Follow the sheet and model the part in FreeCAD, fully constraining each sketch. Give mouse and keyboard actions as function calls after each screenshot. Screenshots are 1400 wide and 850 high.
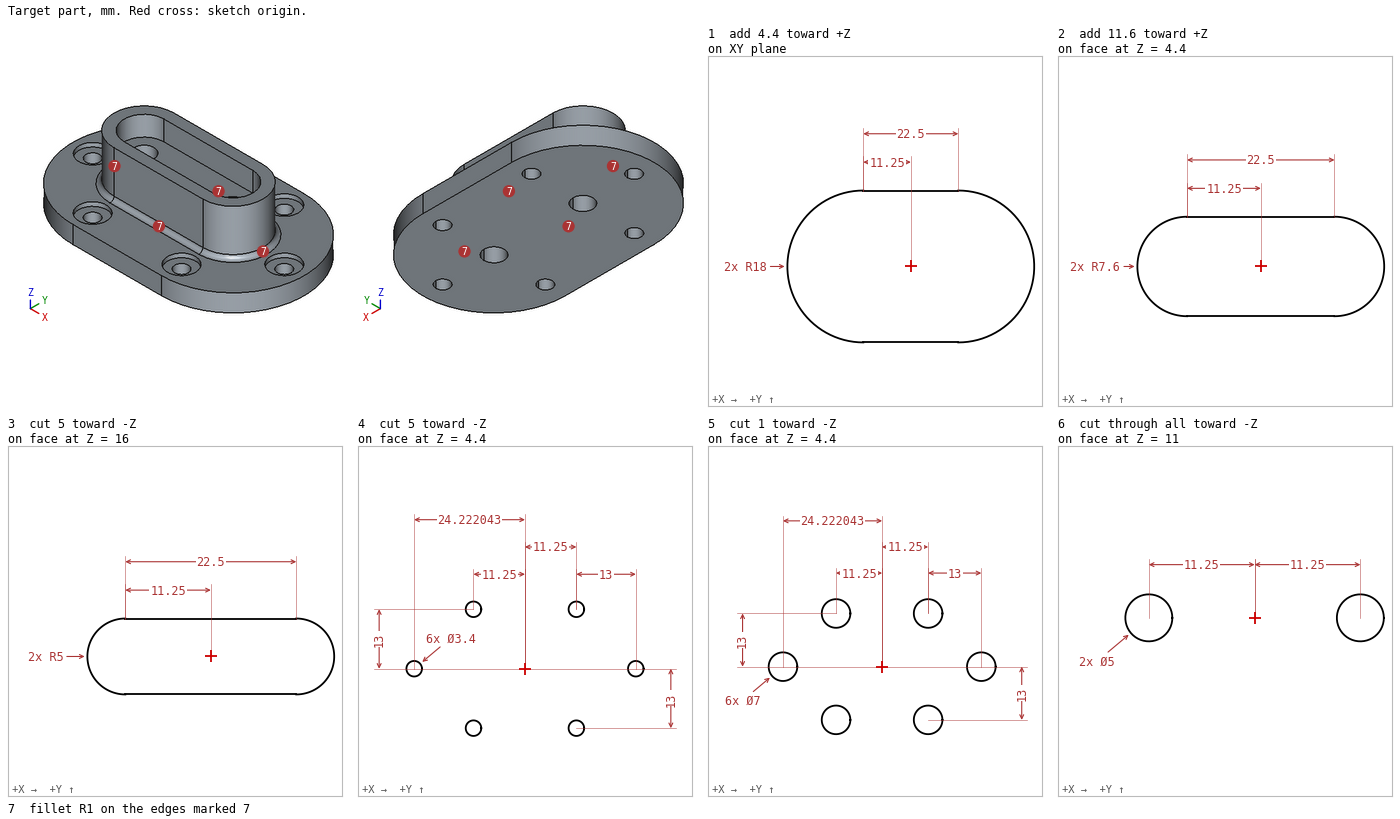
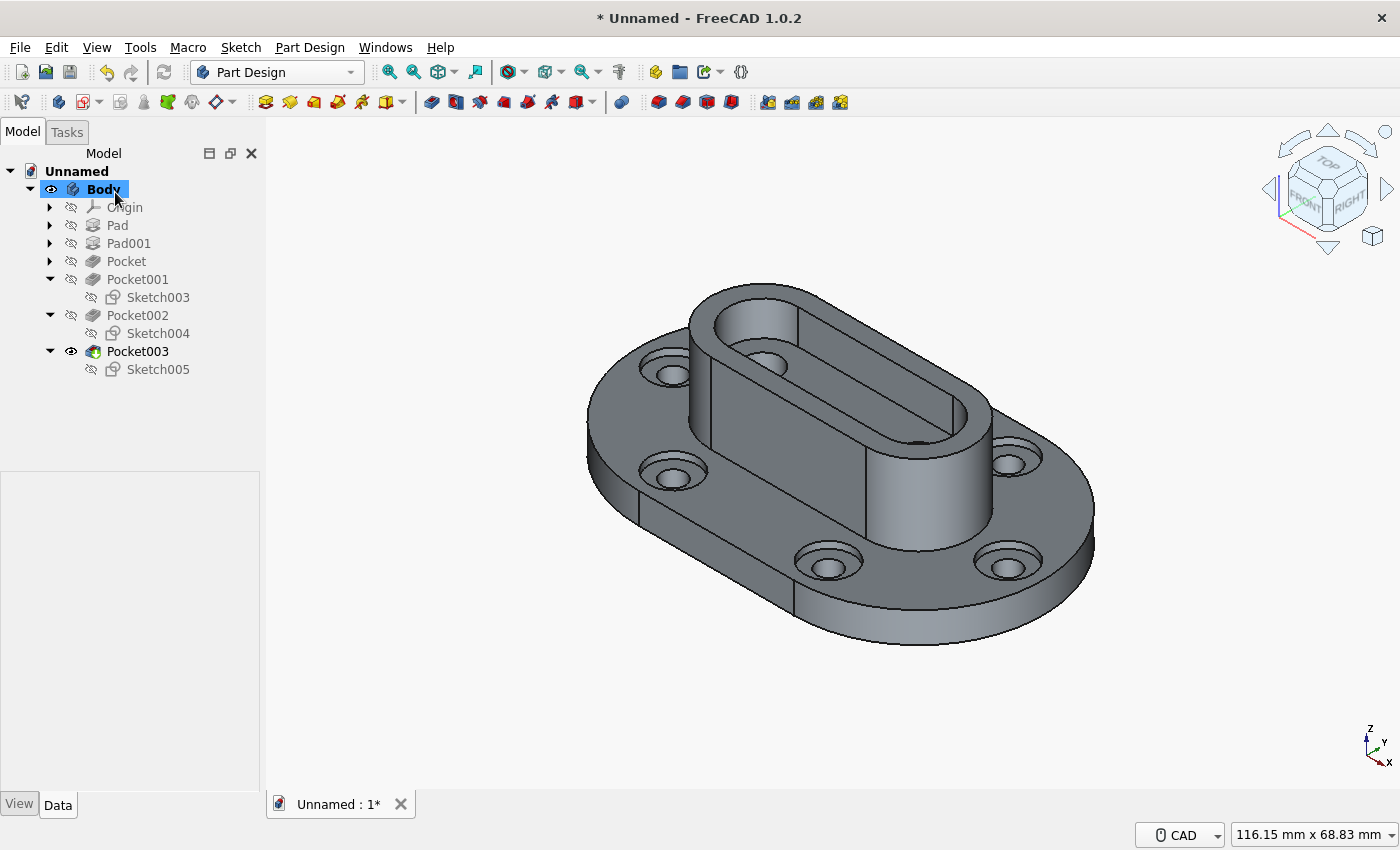
key(2)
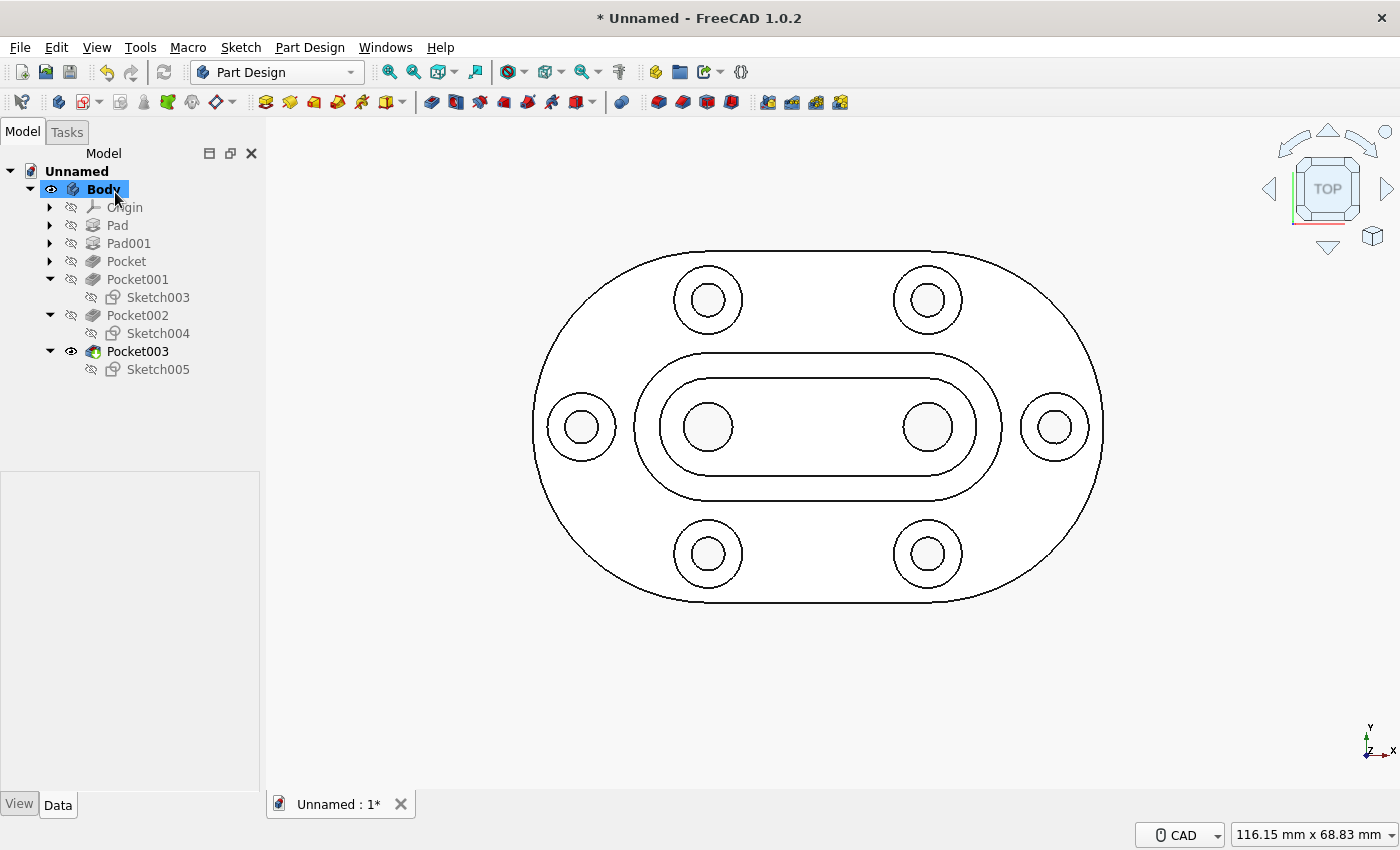
key(1)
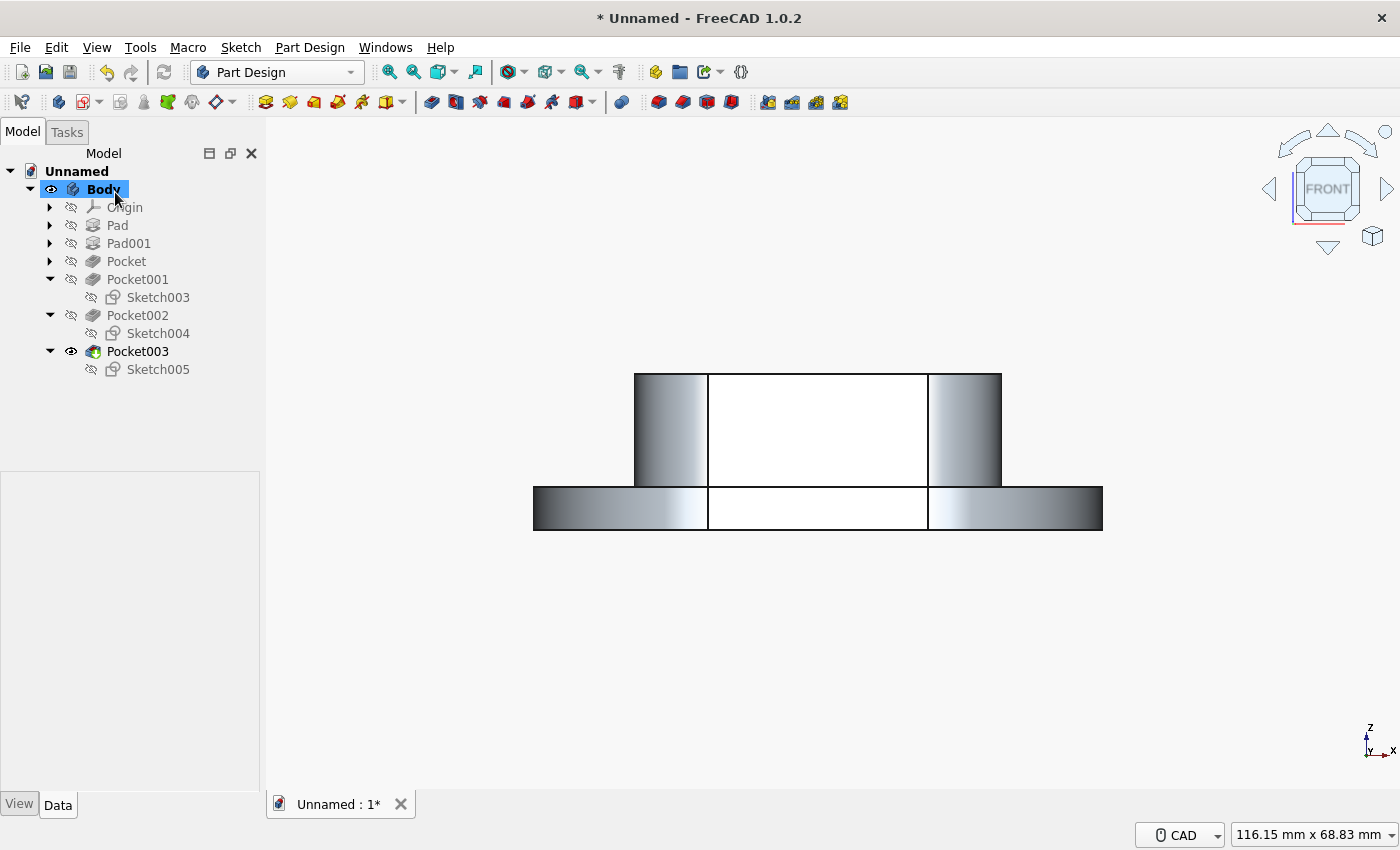
key(3)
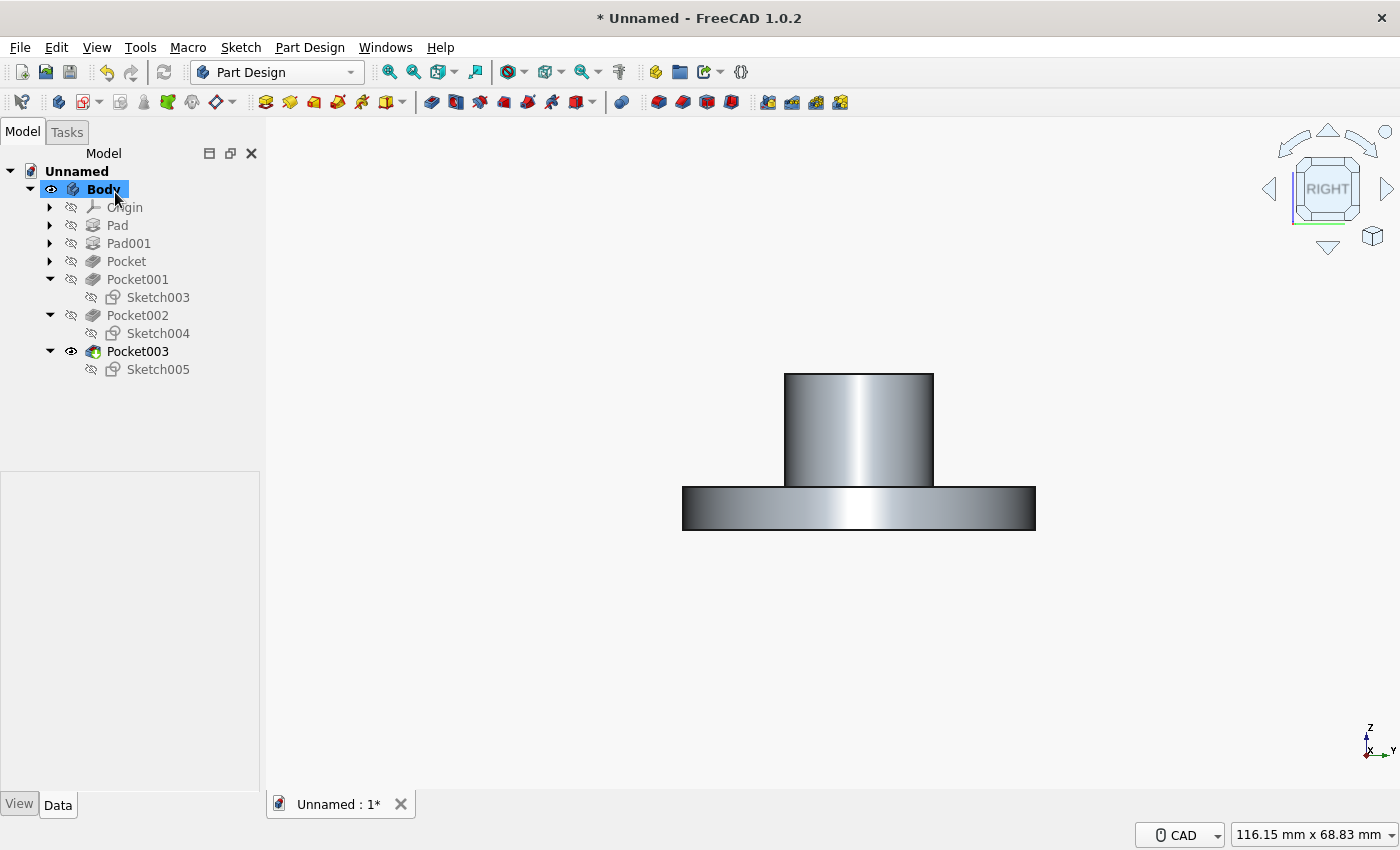
click(390, 72)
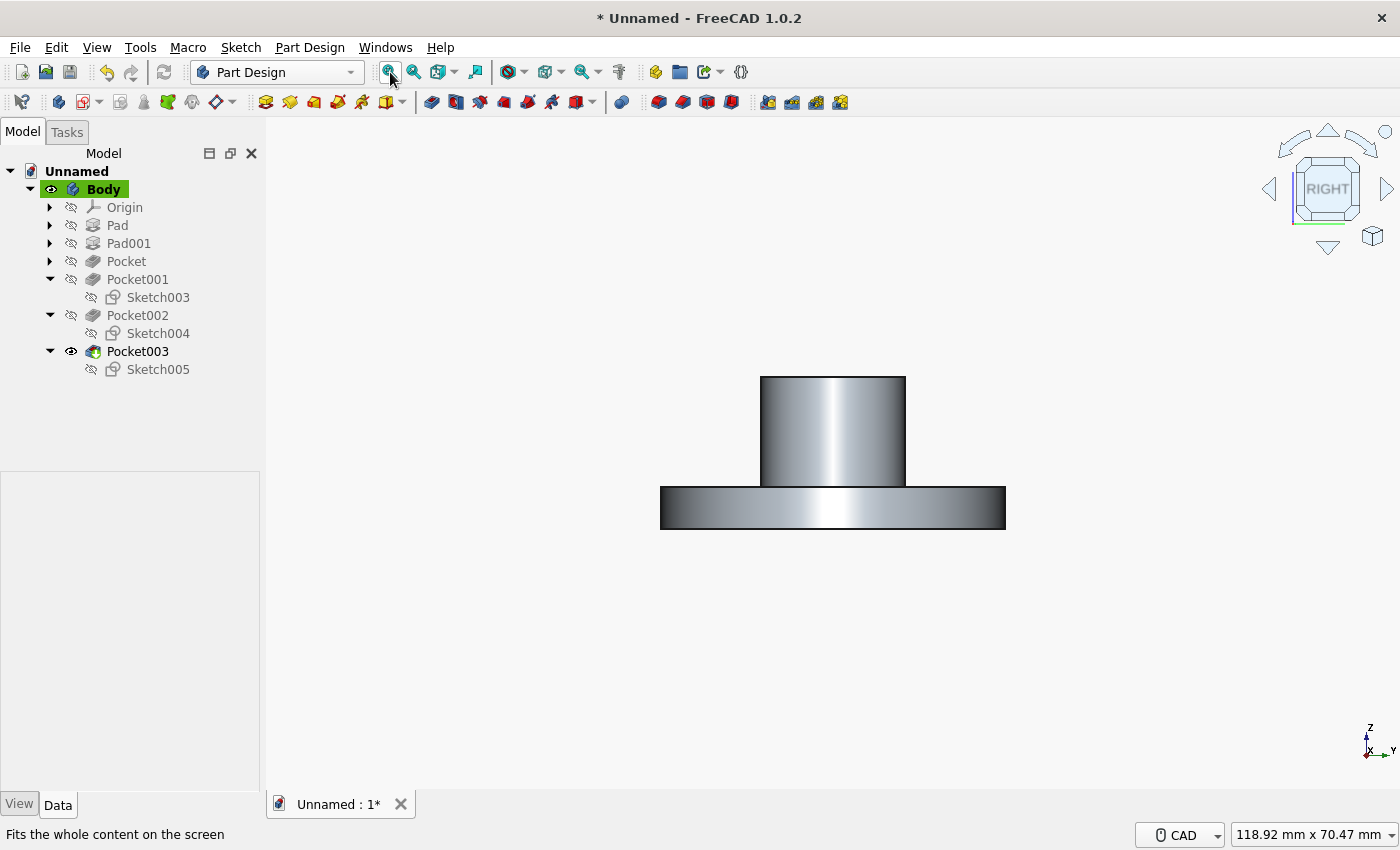
key(5)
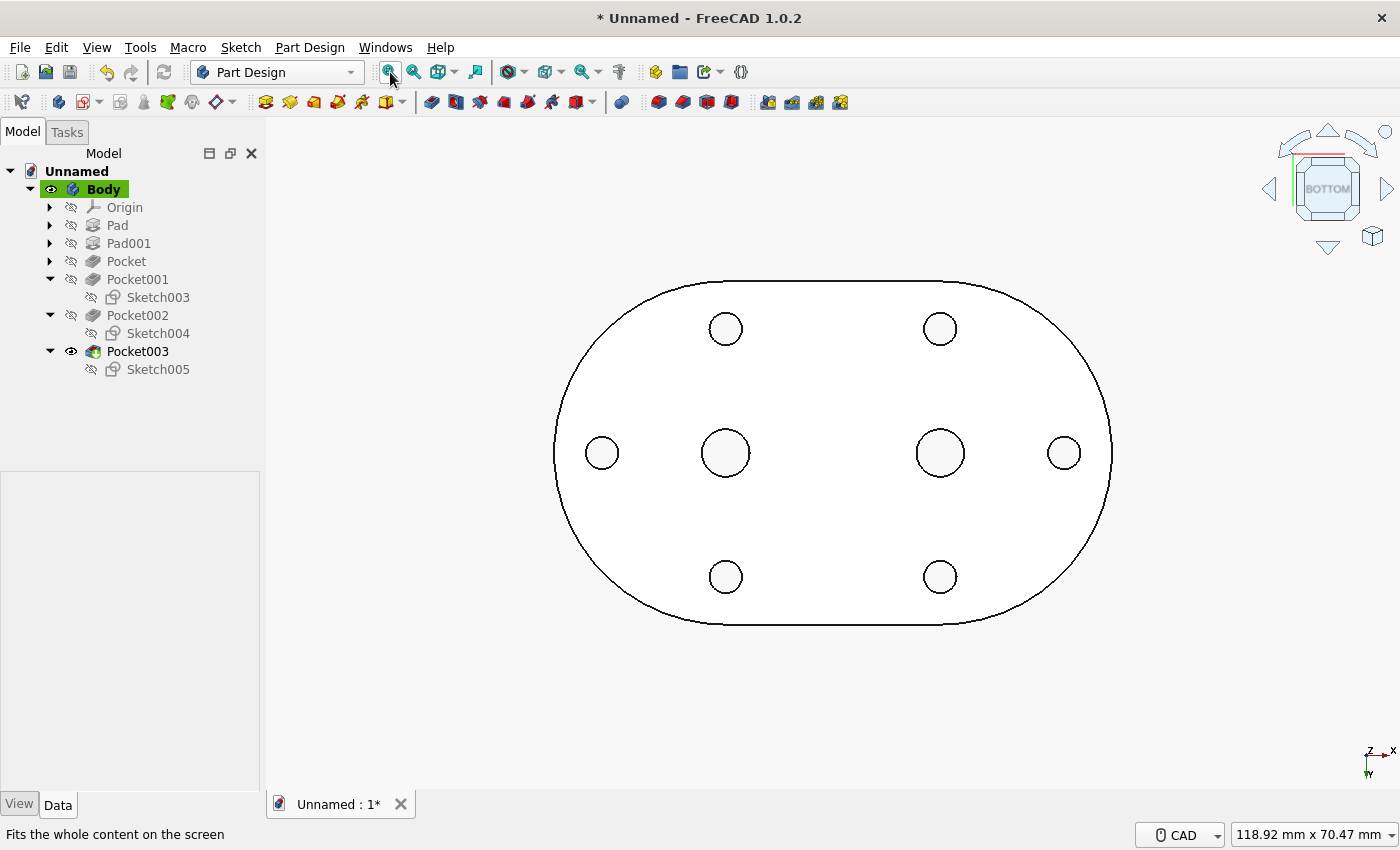
key(4)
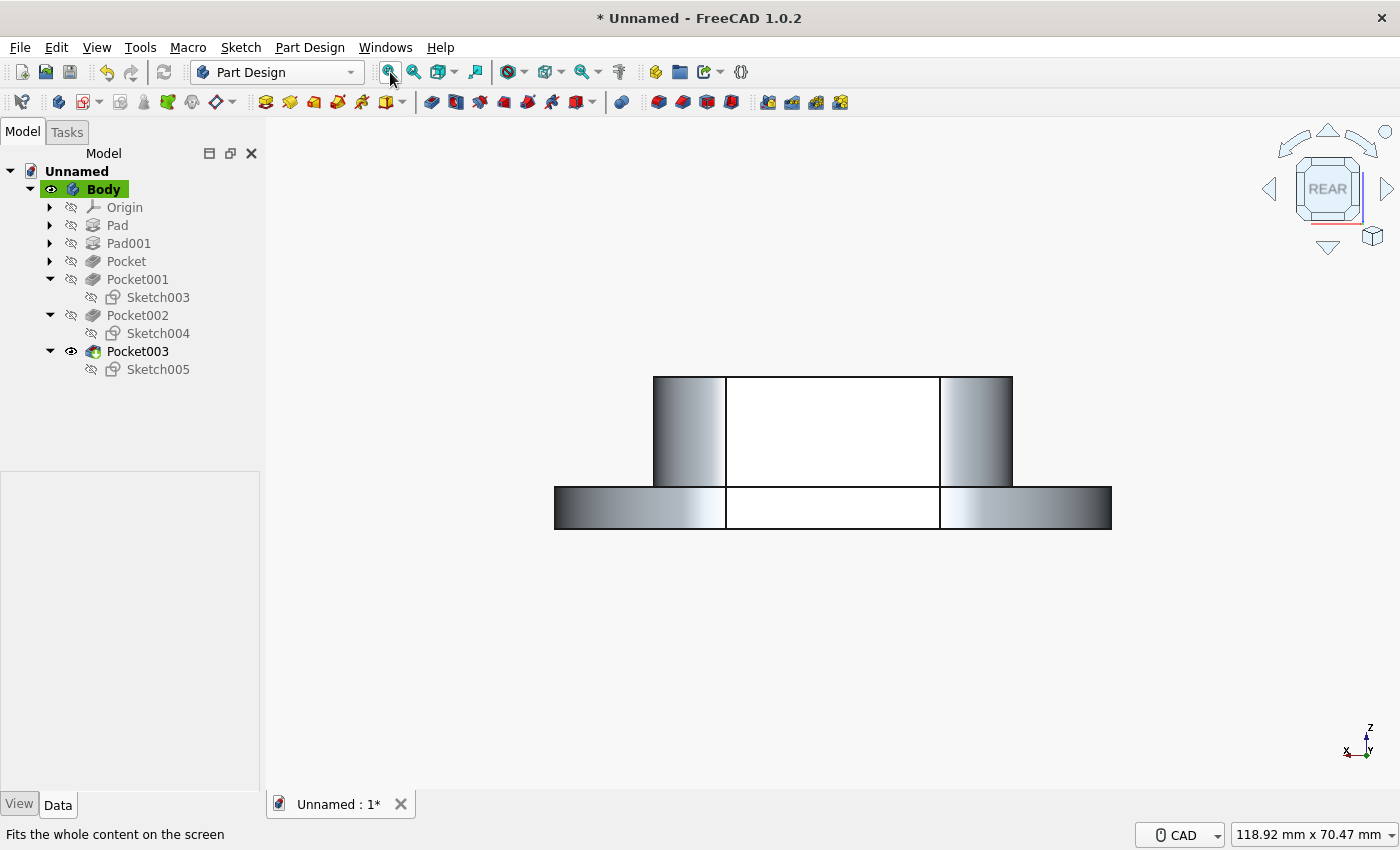
key(6)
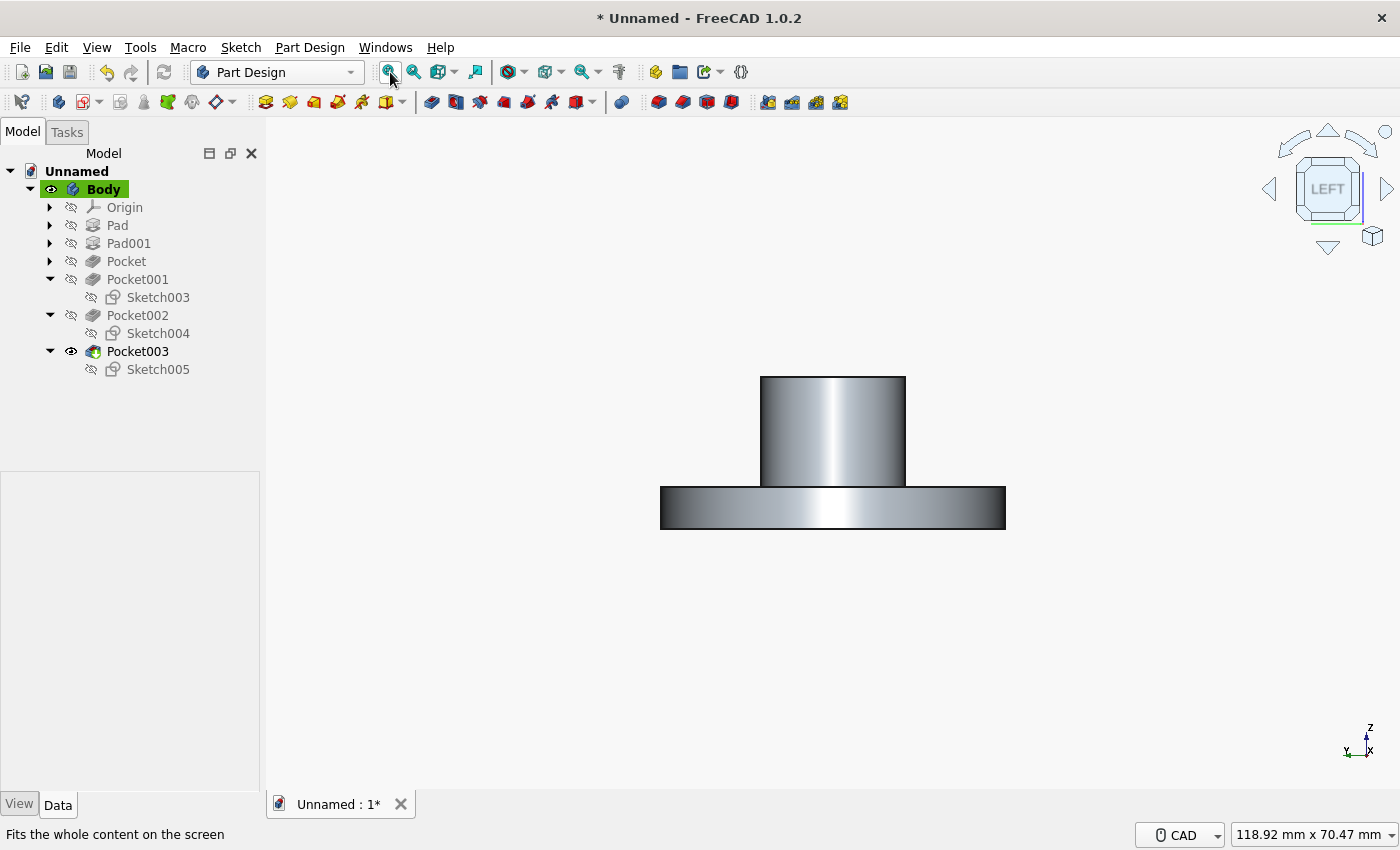
click(390, 72)